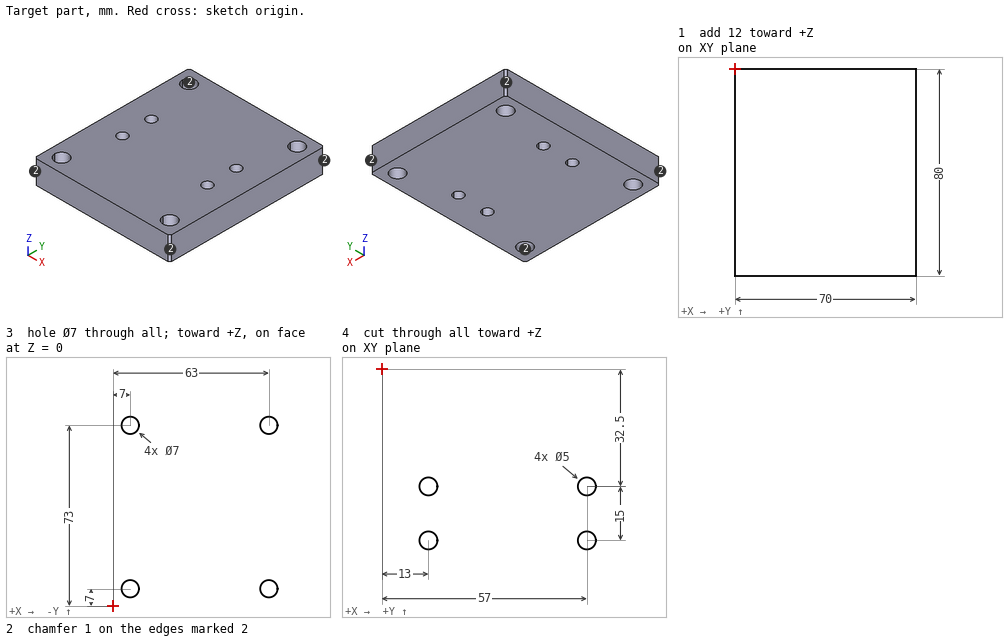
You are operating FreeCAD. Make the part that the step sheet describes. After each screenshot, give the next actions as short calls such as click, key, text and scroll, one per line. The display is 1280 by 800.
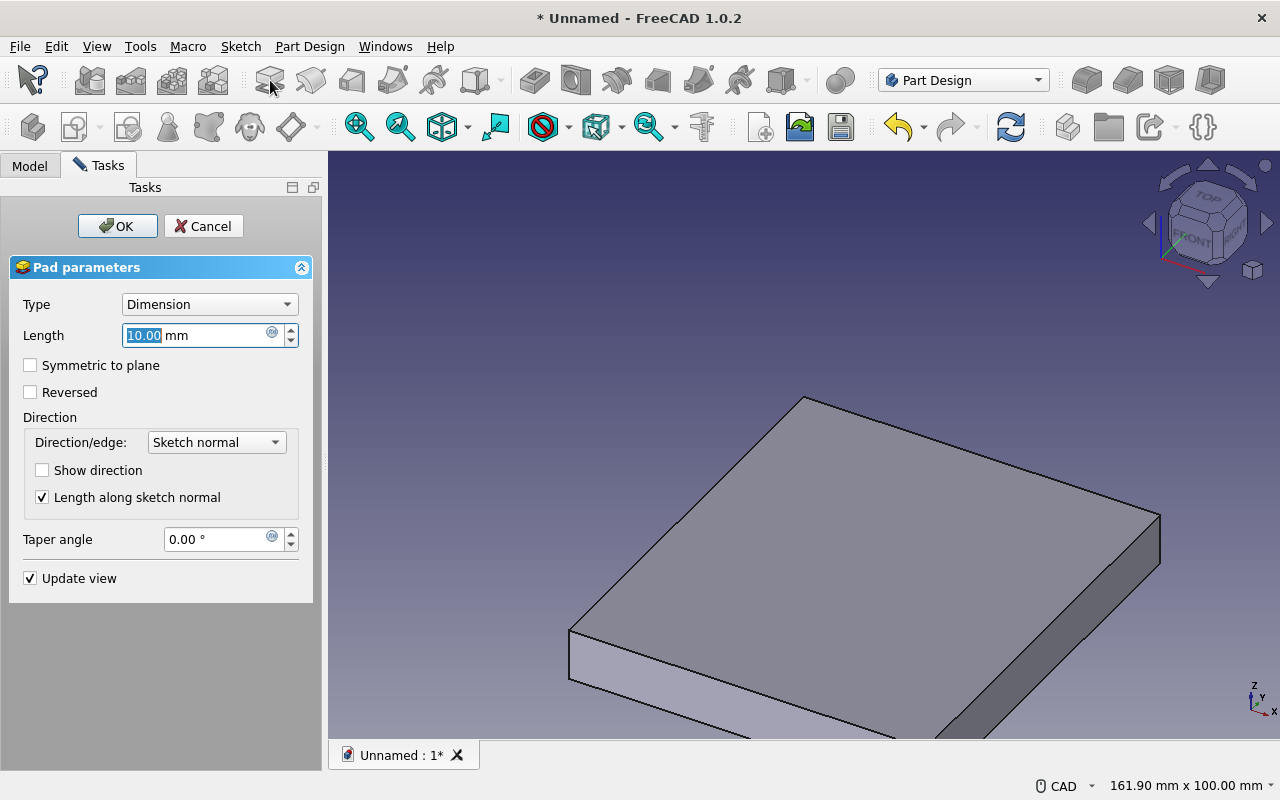
text(12)
key(Tab)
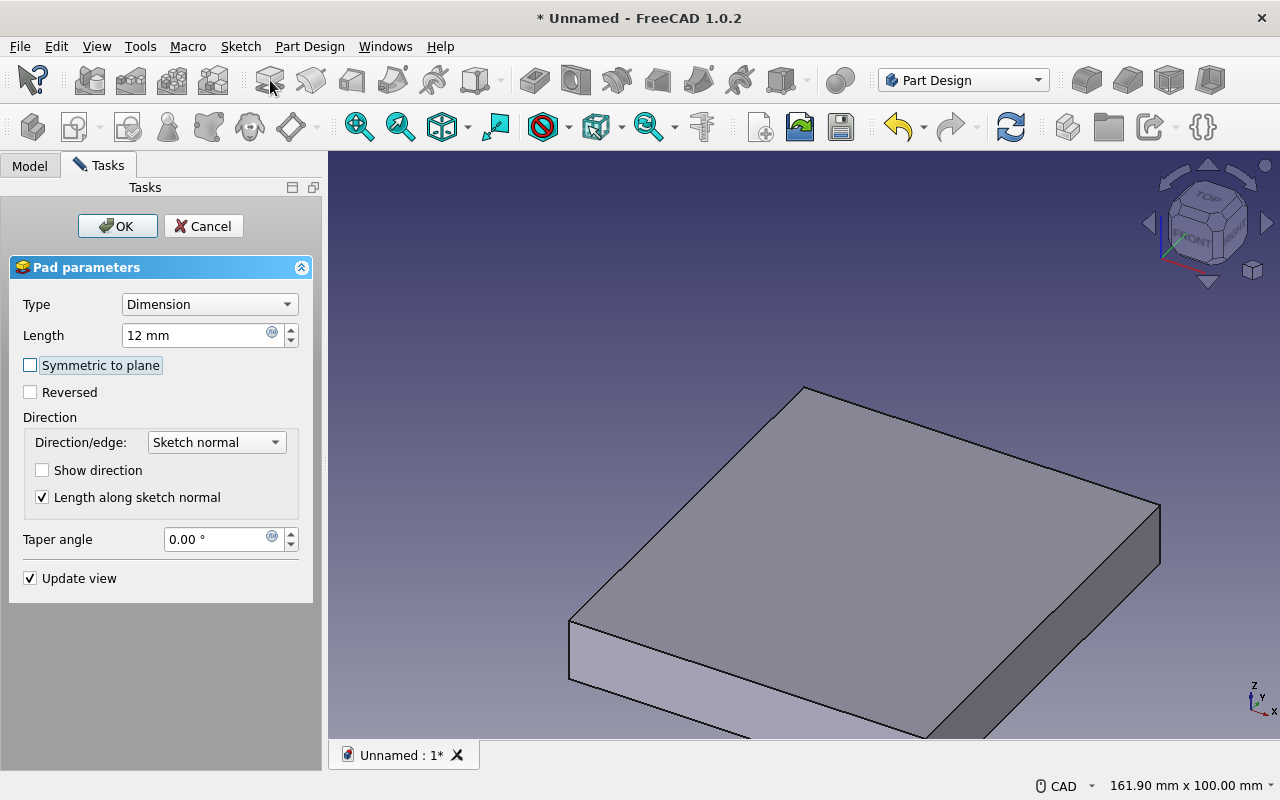
click(118, 226)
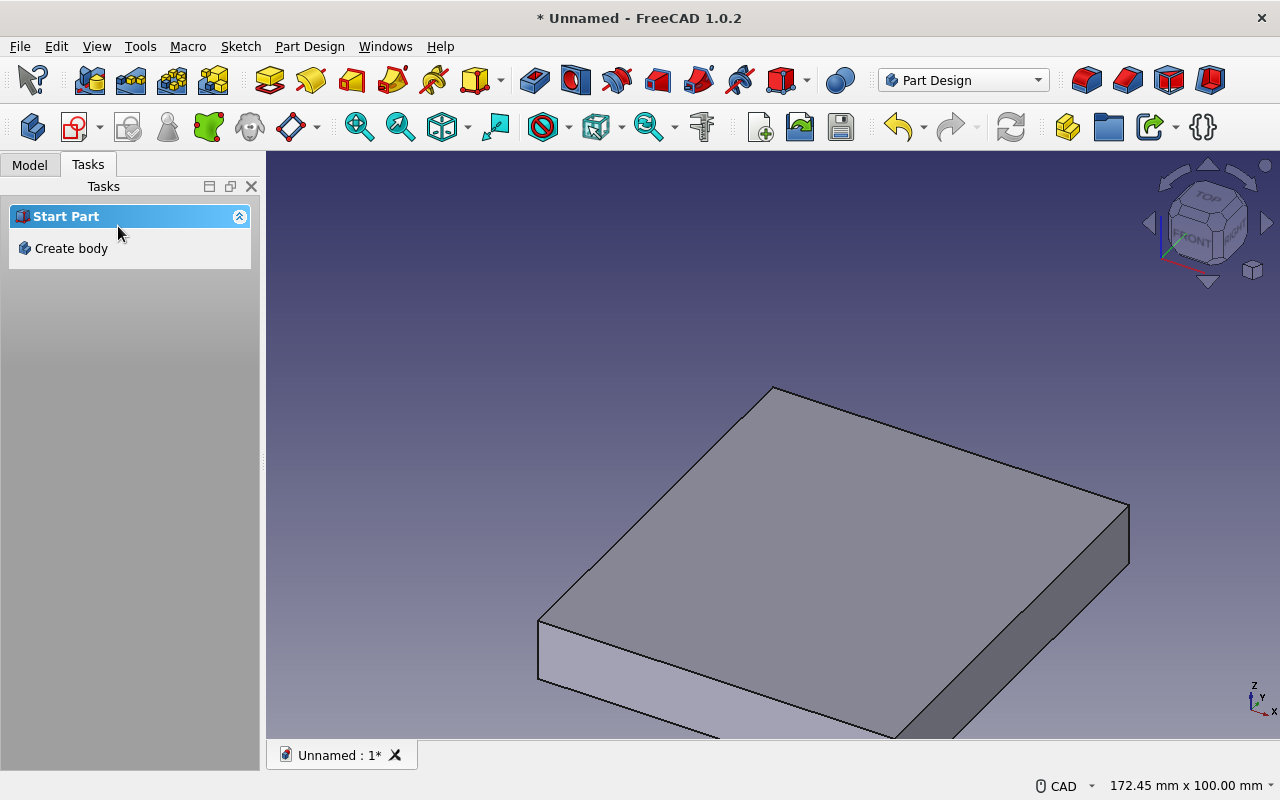
click(360, 128)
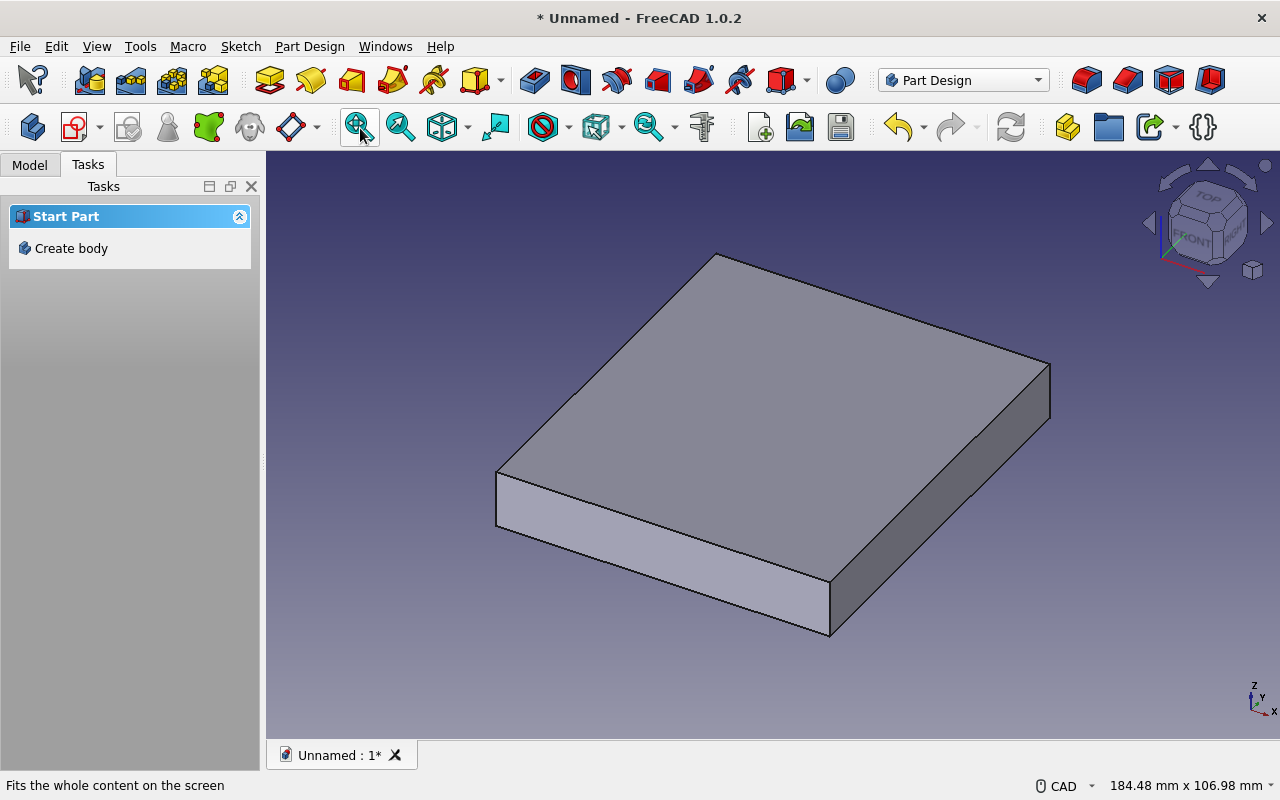
click(830, 608)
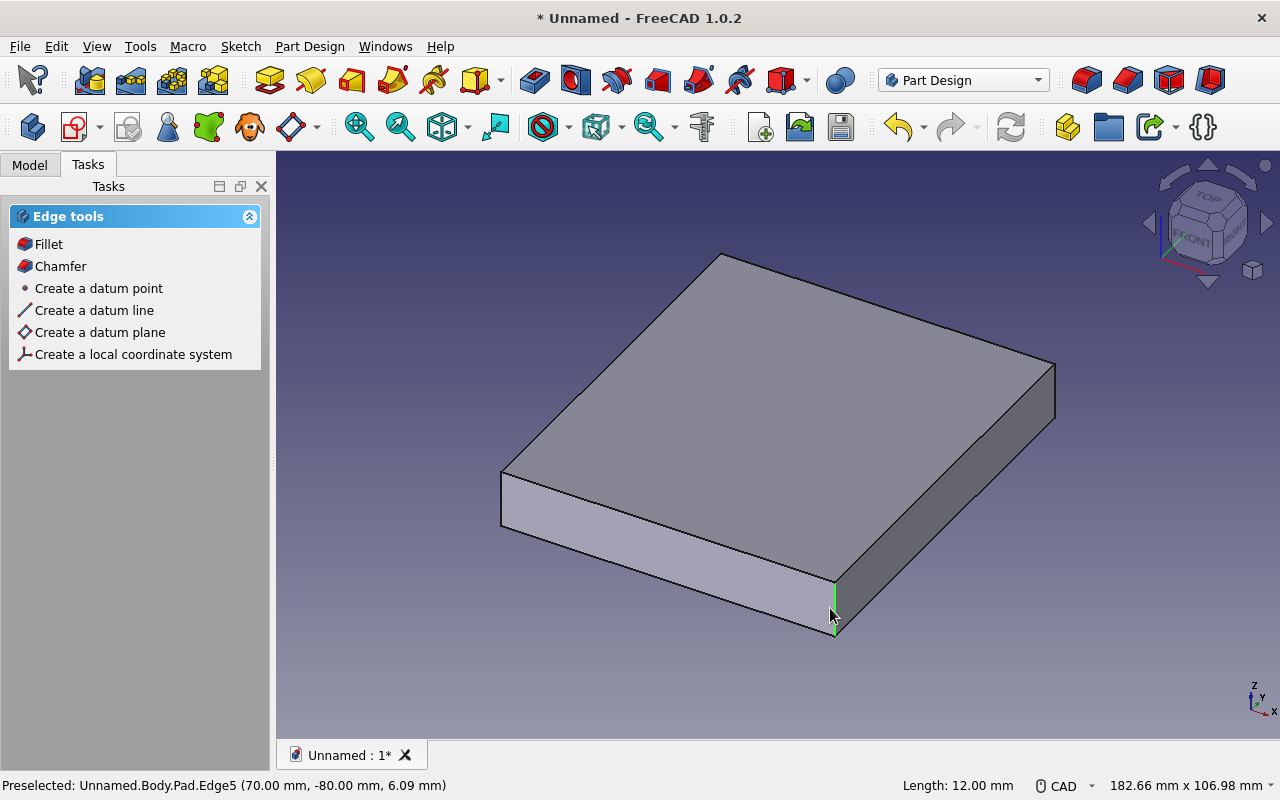
key(0)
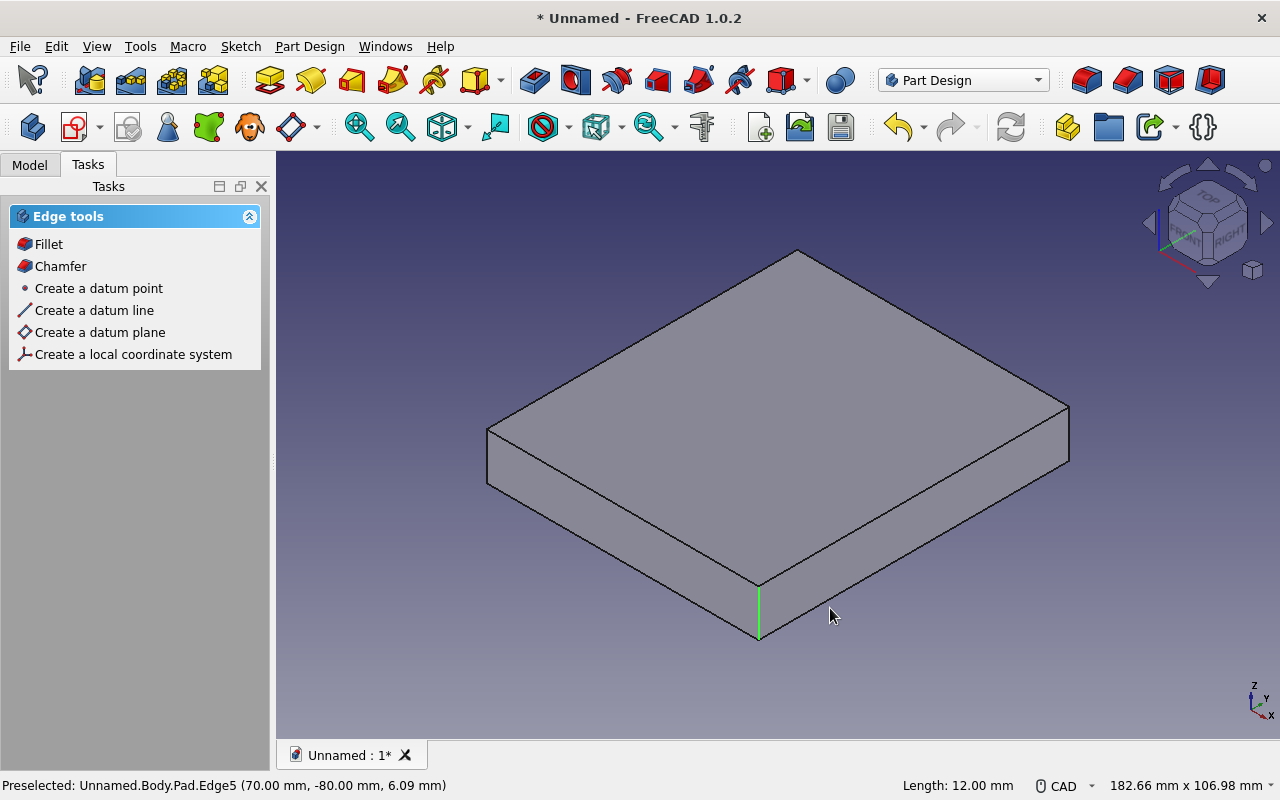
key(2)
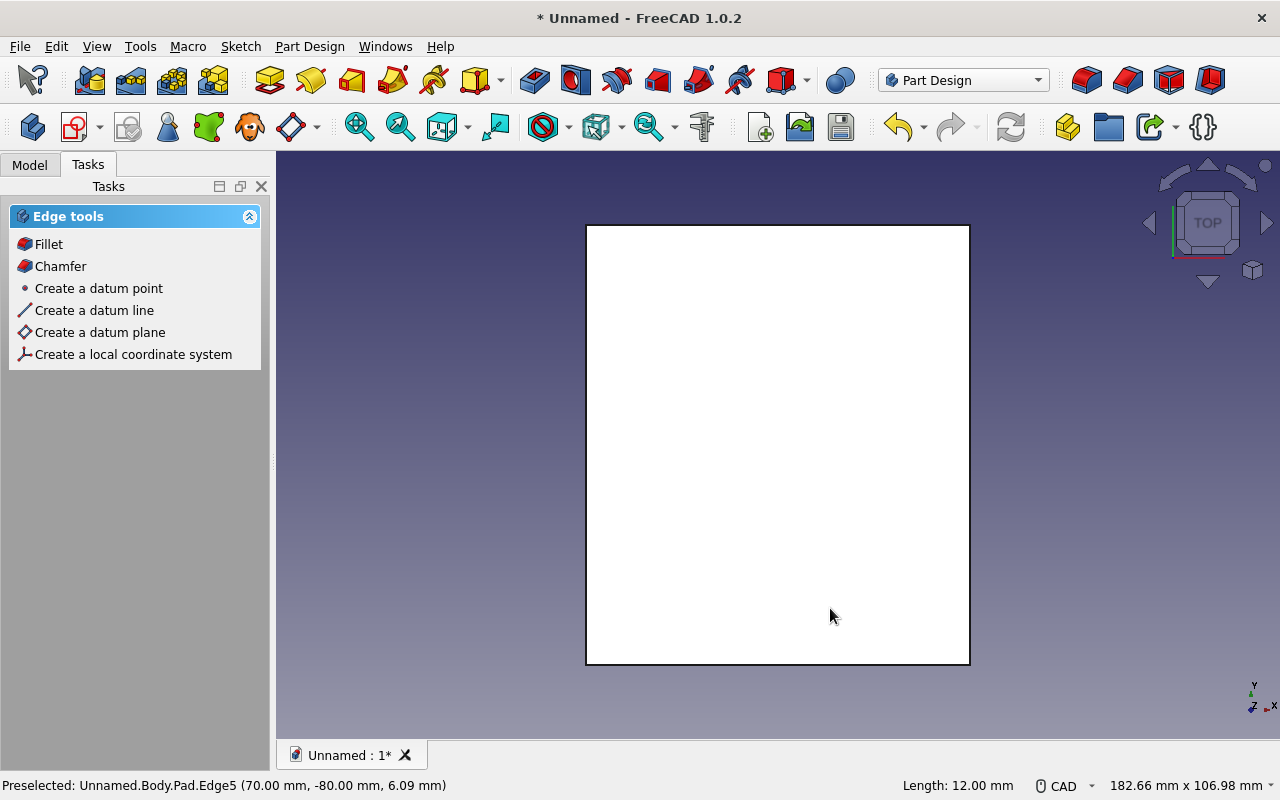
key(1)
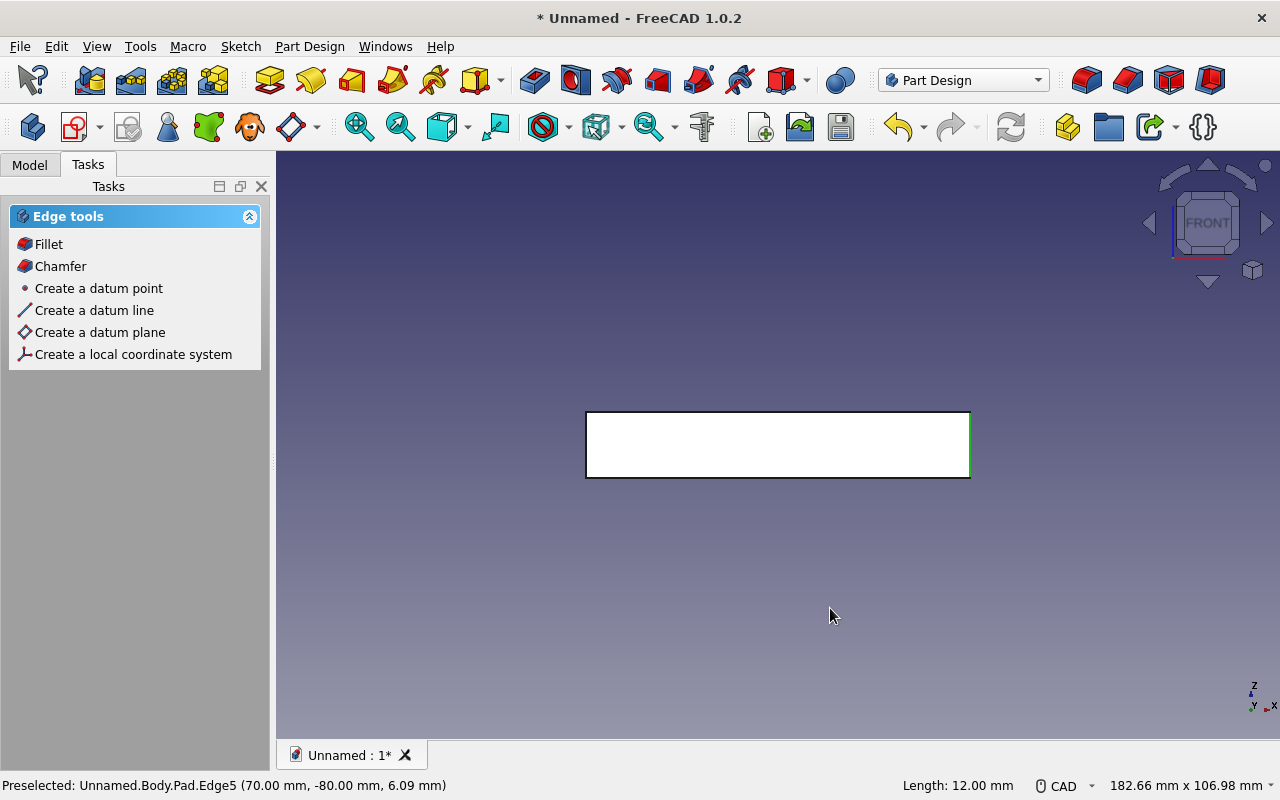
click(360, 128)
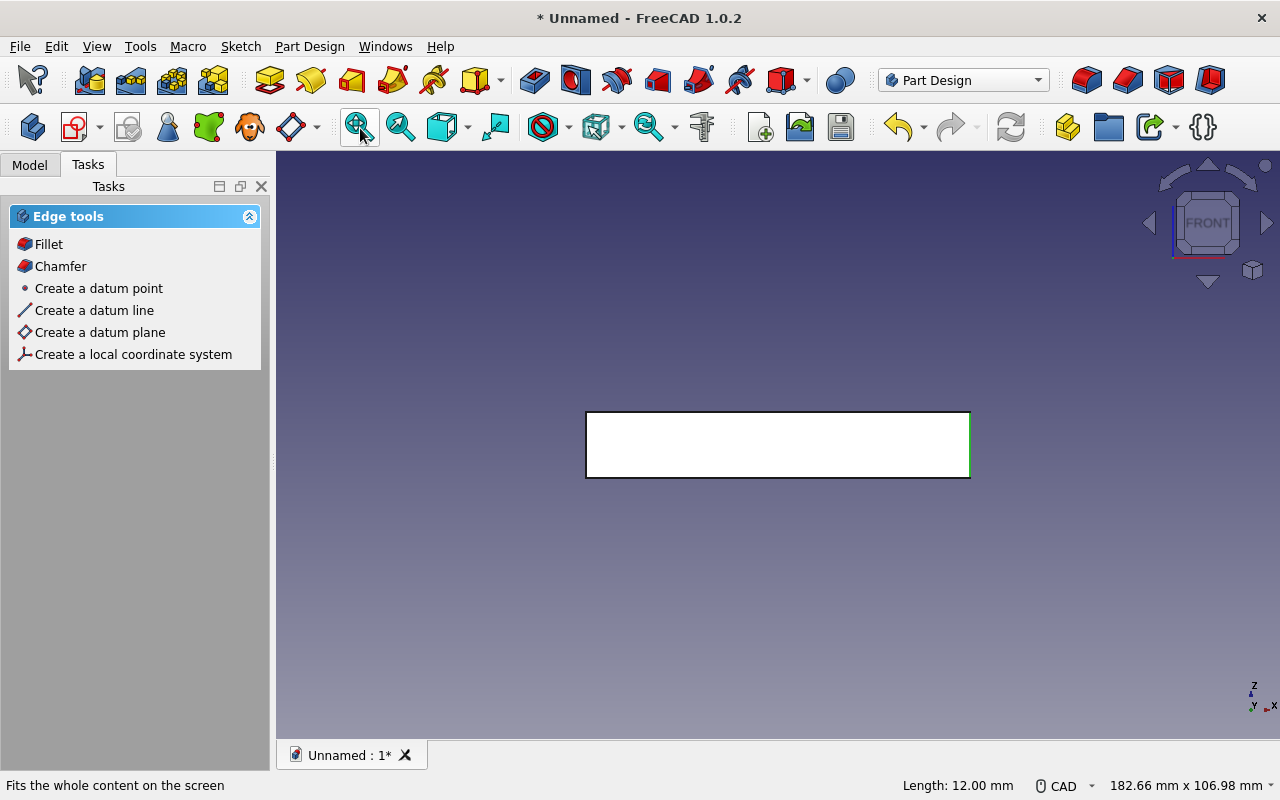
click(586, 444, ctrl)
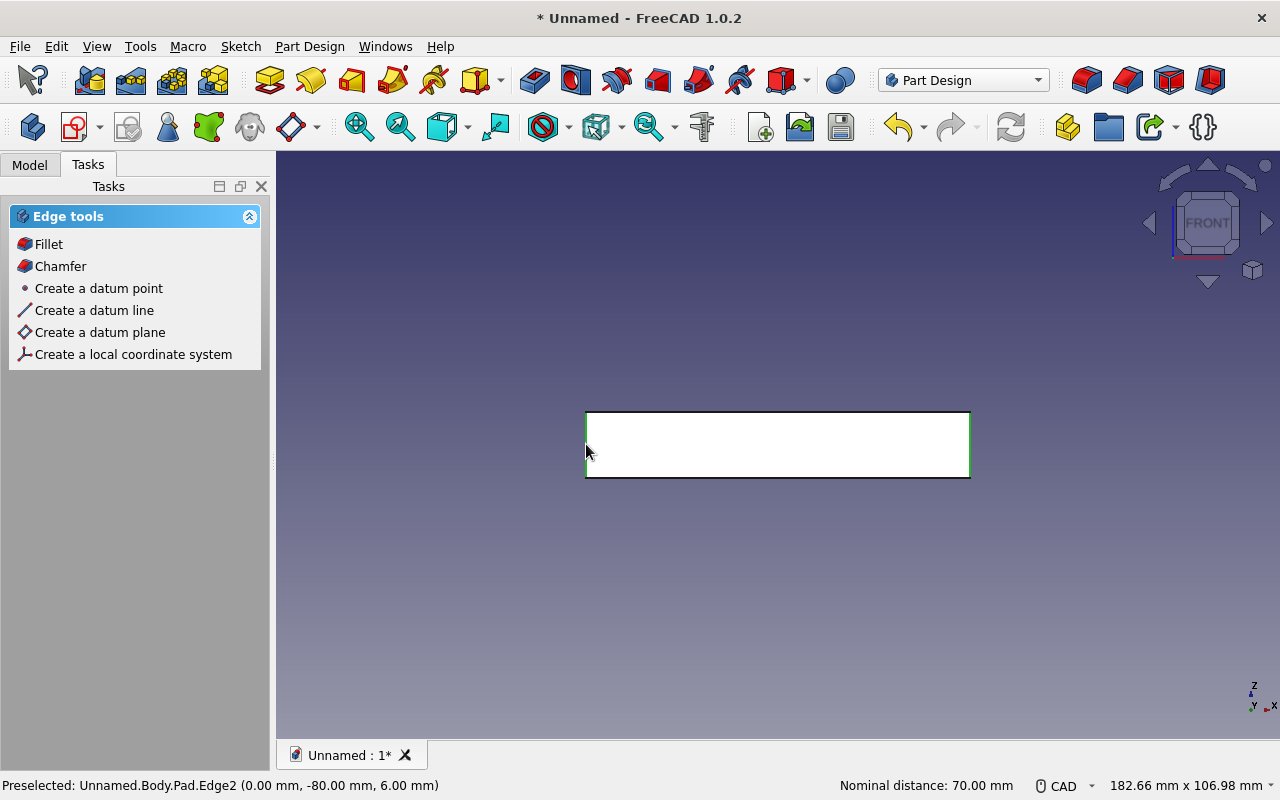
key(3)